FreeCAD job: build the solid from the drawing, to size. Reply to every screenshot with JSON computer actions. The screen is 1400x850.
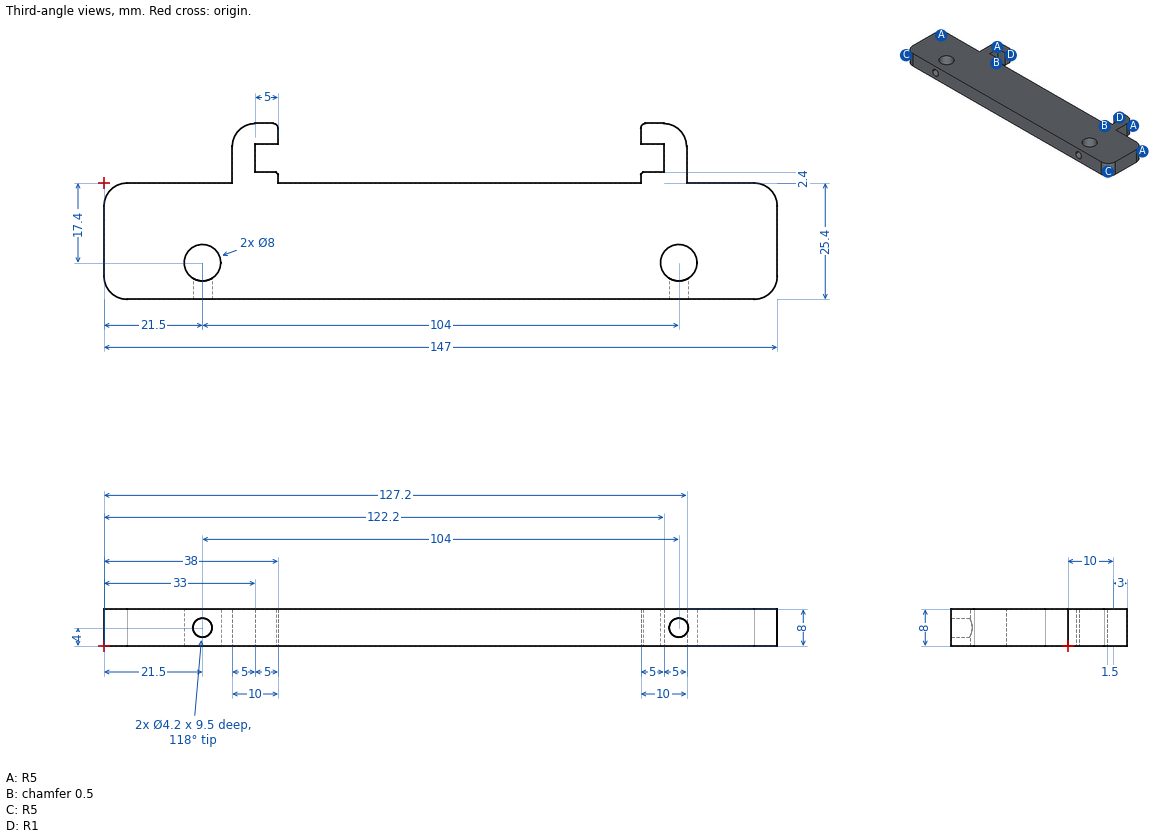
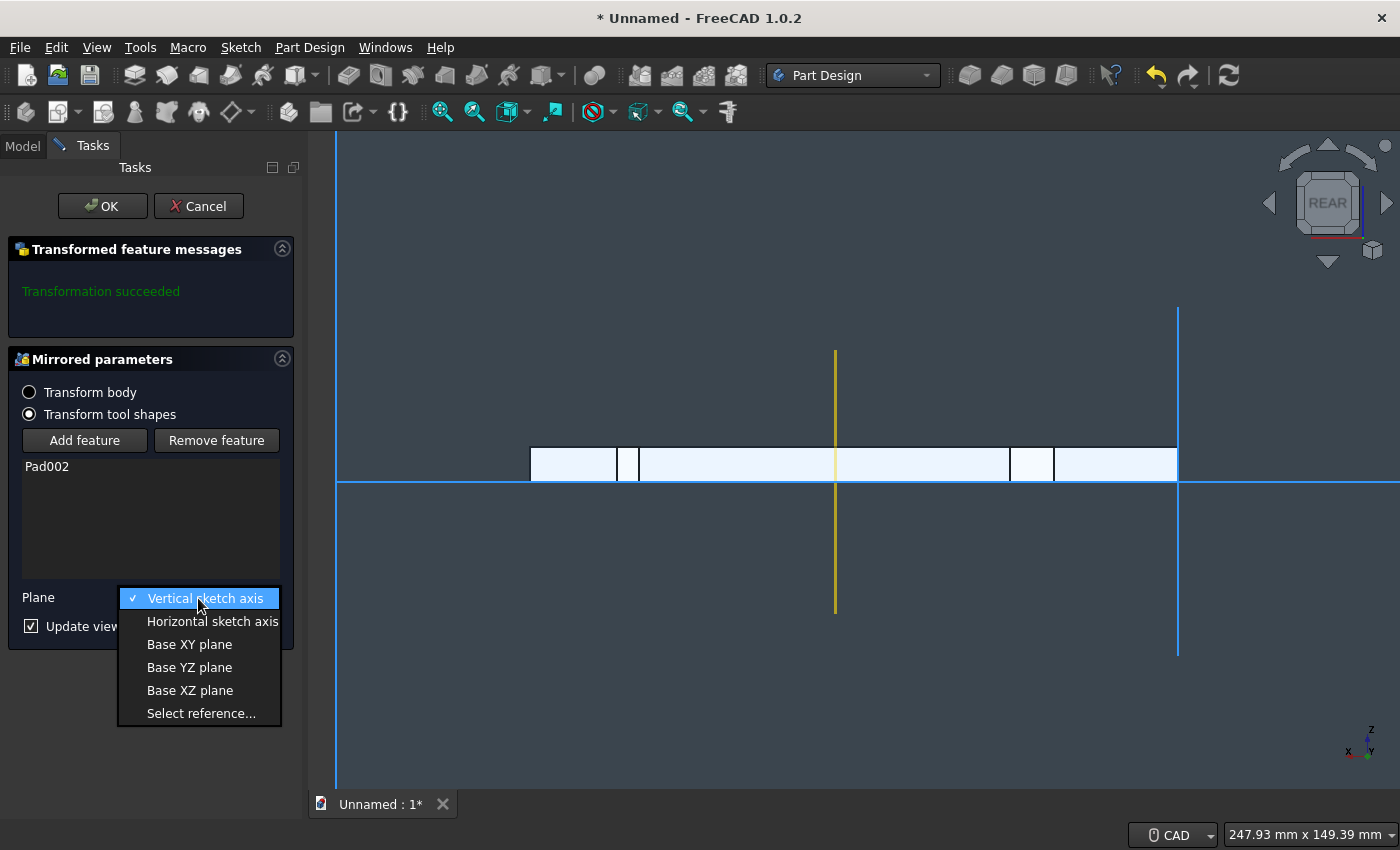
{"action": "left_click", "coordinate": [198, 714]}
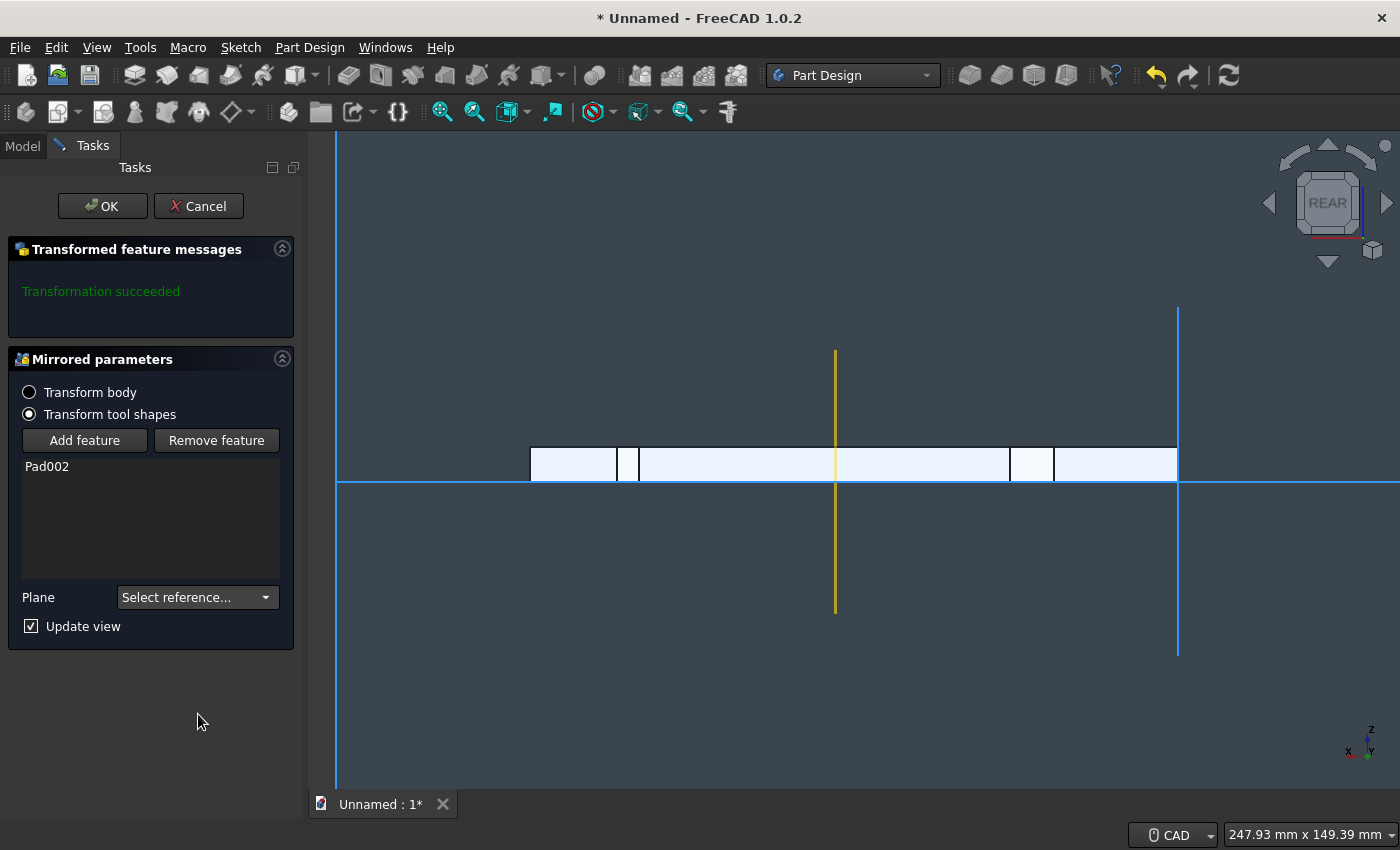
{"action": "left_click", "coordinate": [23, 145]}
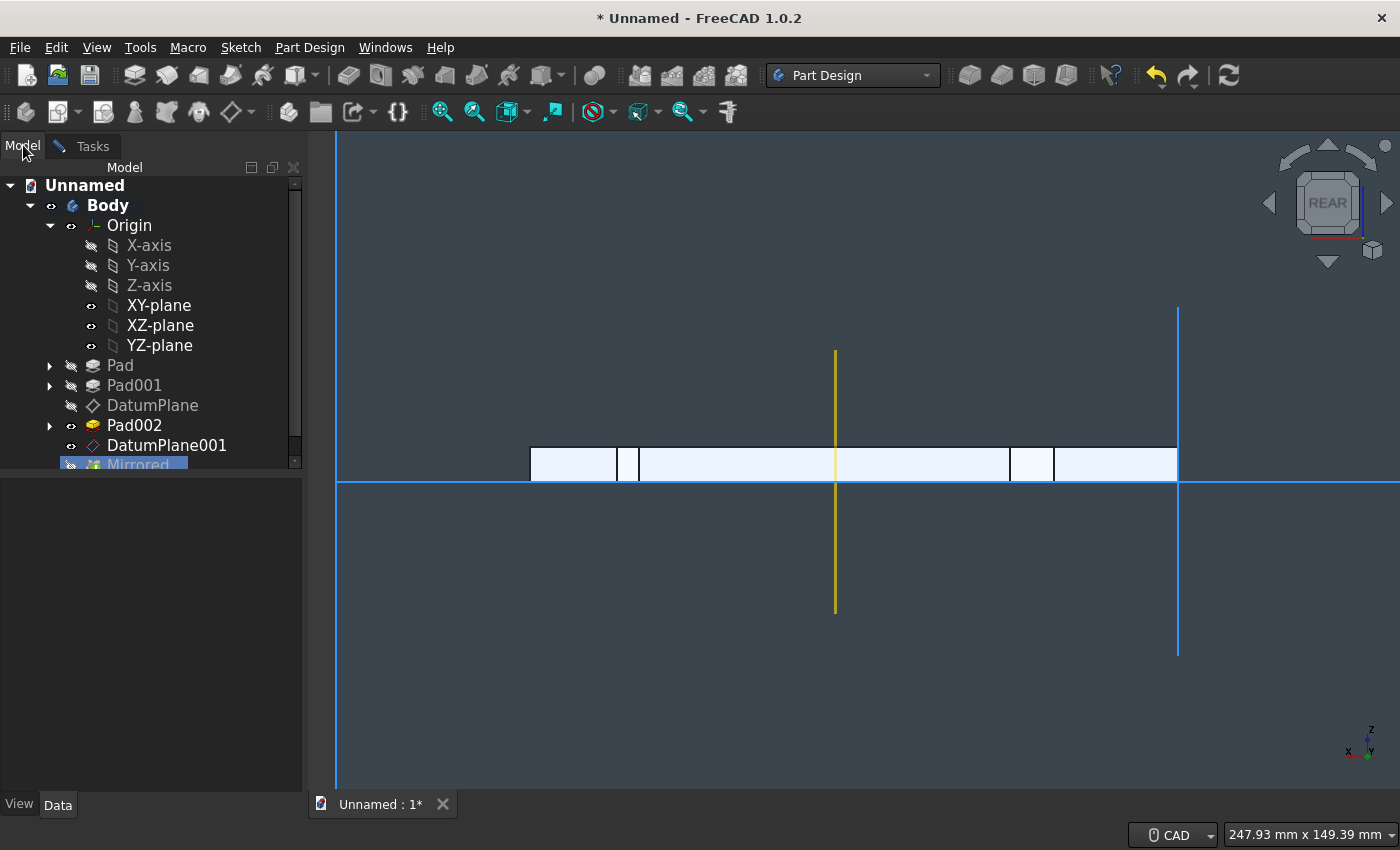
{"action": "left_click", "coordinate": [116, 446]}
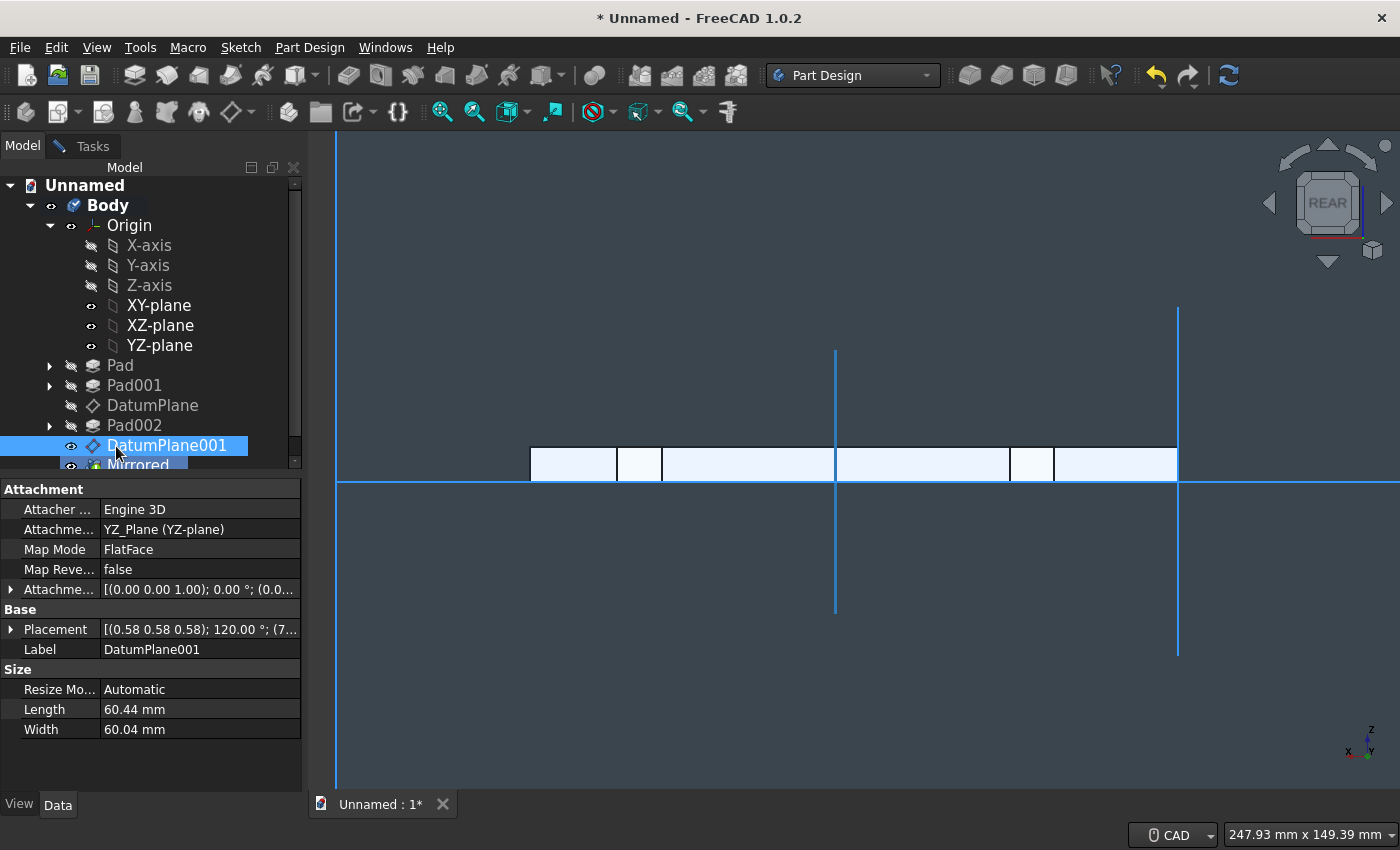
{"action": "left_click", "coordinate": [84, 145]}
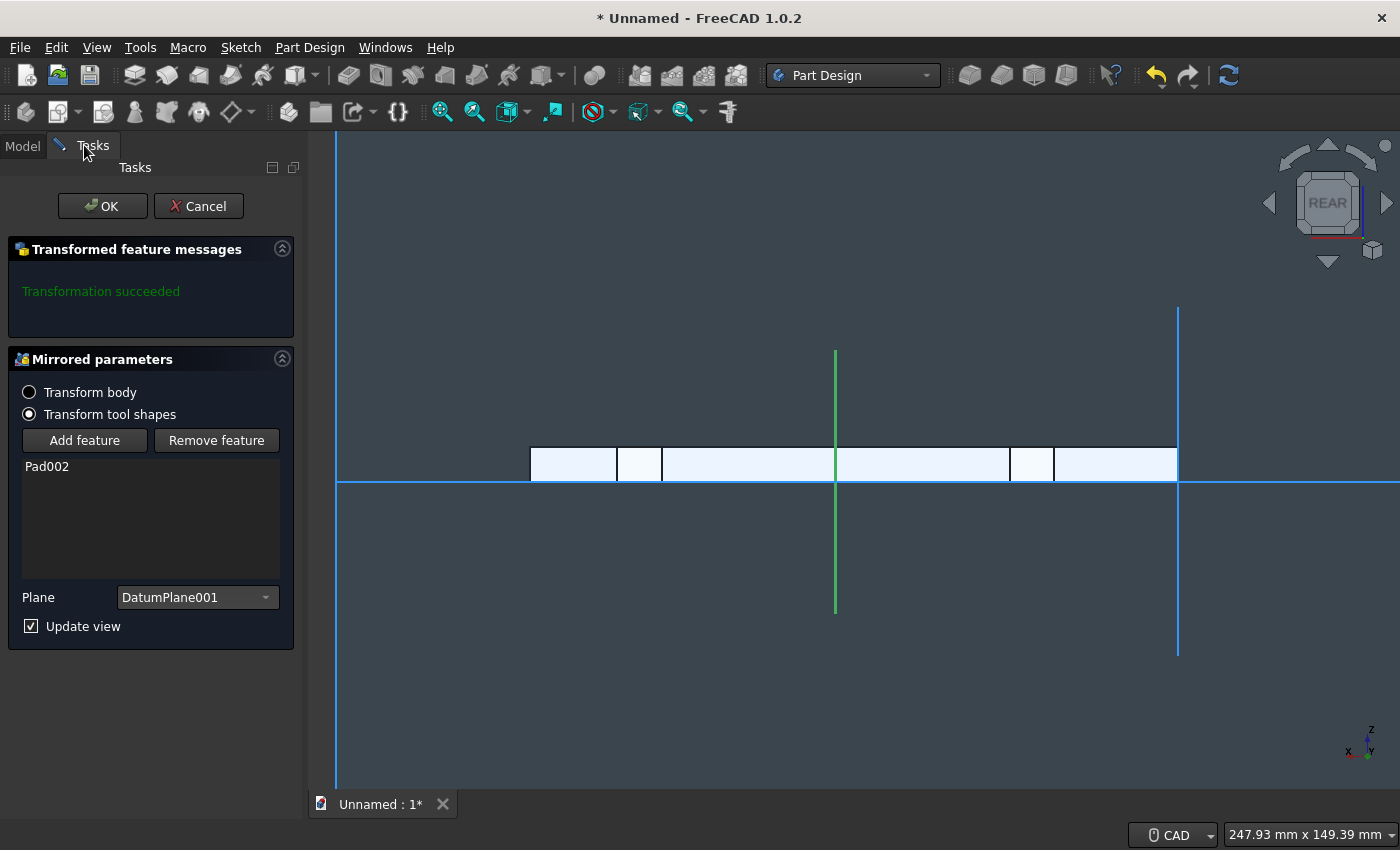
{"action": "left_click", "coordinate": [103, 206]}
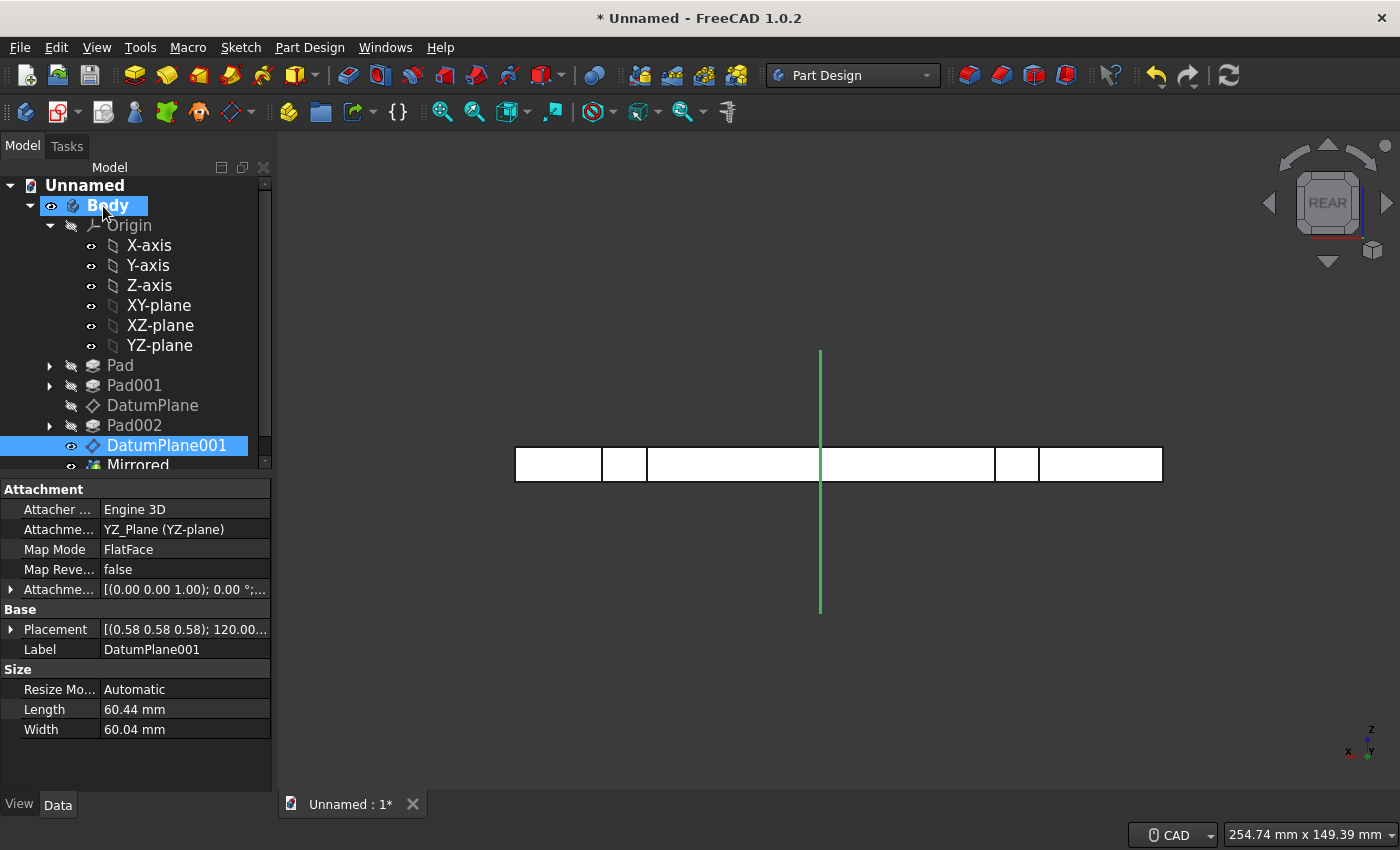
{"action": "left_click", "coordinate": [116, 446]}
{"action": "key", "text": "space"}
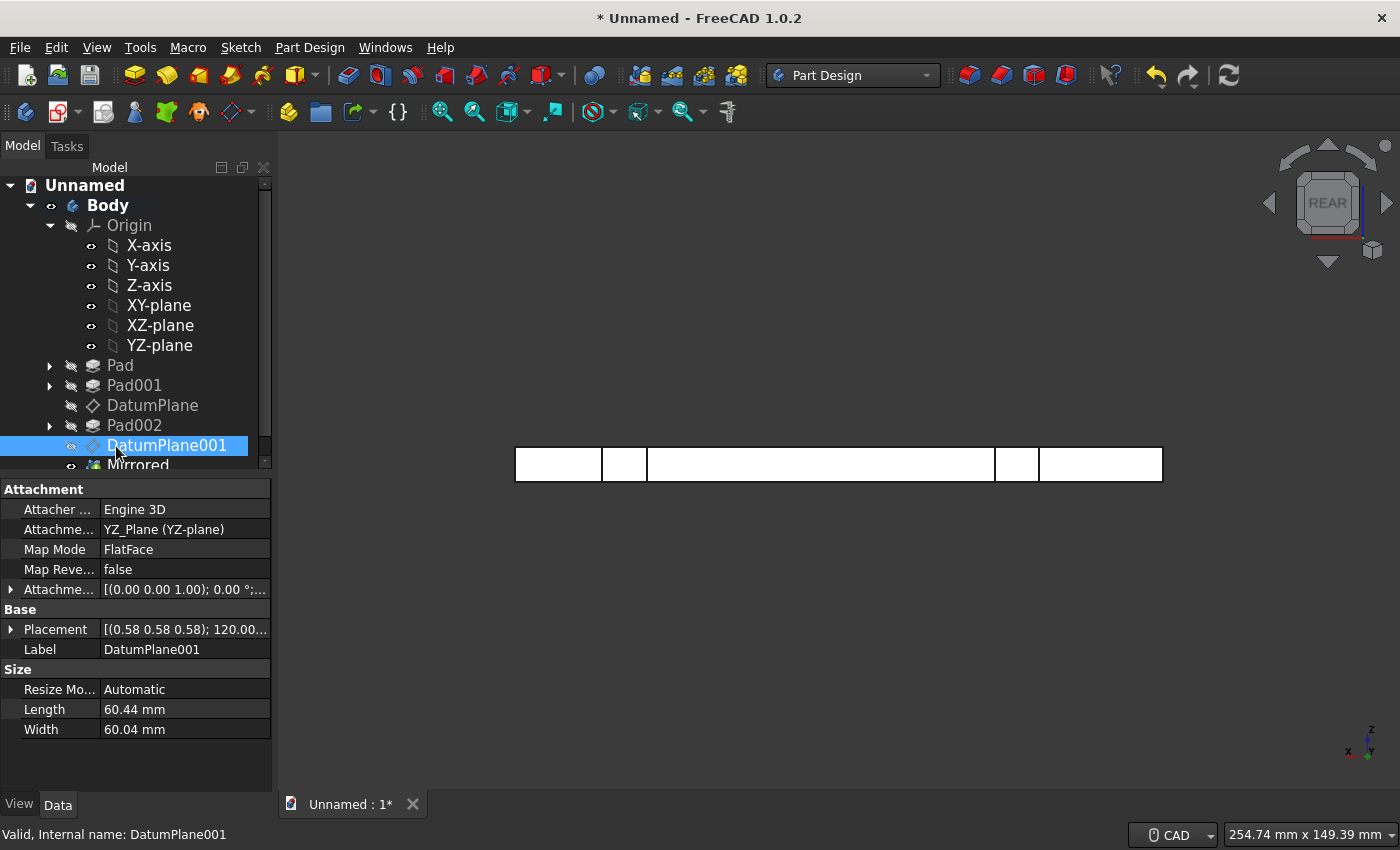
{"action": "left_click", "coordinate": [709, 463]}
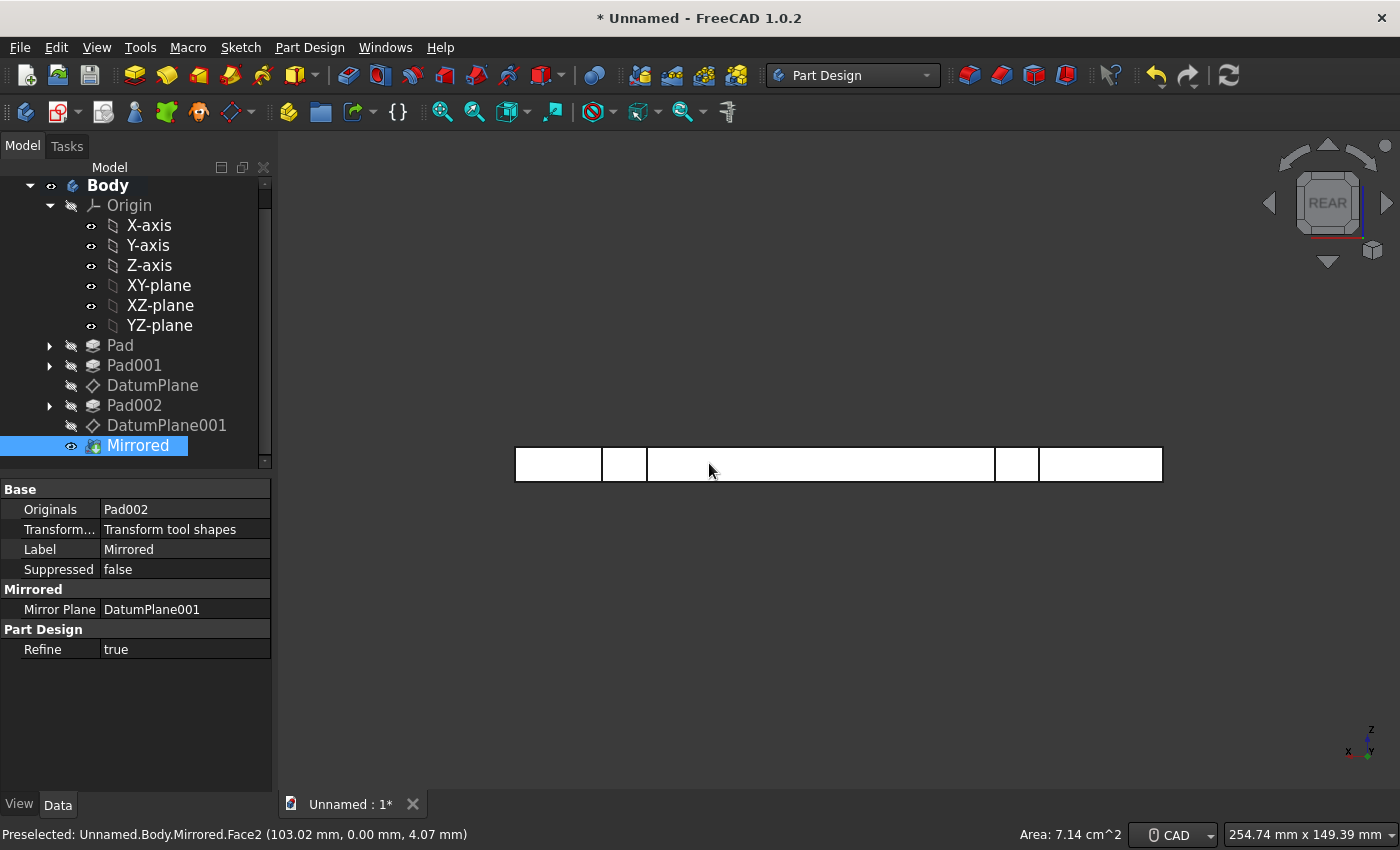
{"action": "left_click", "coordinate": [58, 112]}